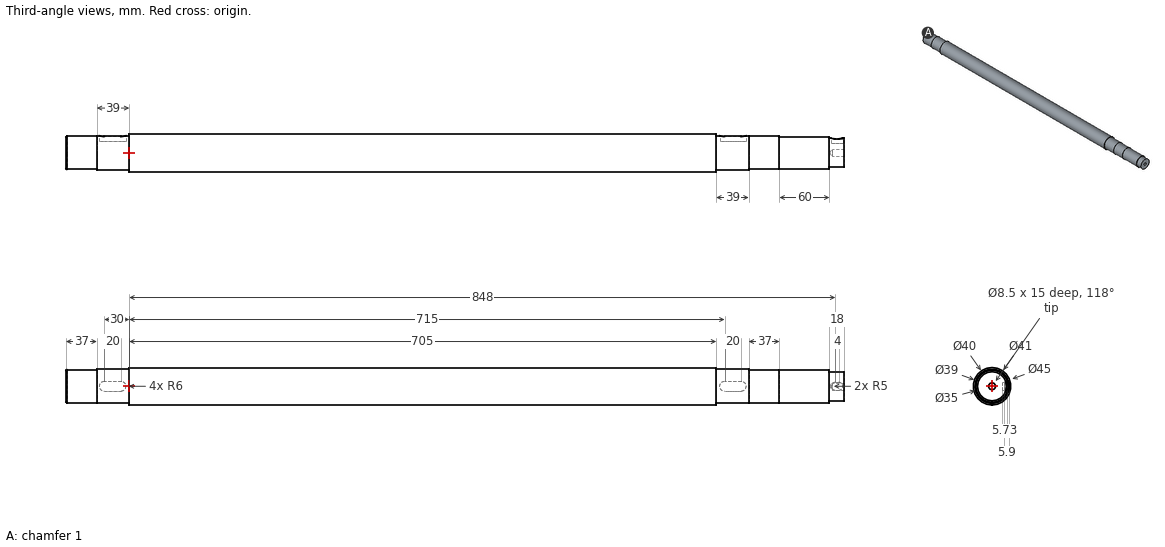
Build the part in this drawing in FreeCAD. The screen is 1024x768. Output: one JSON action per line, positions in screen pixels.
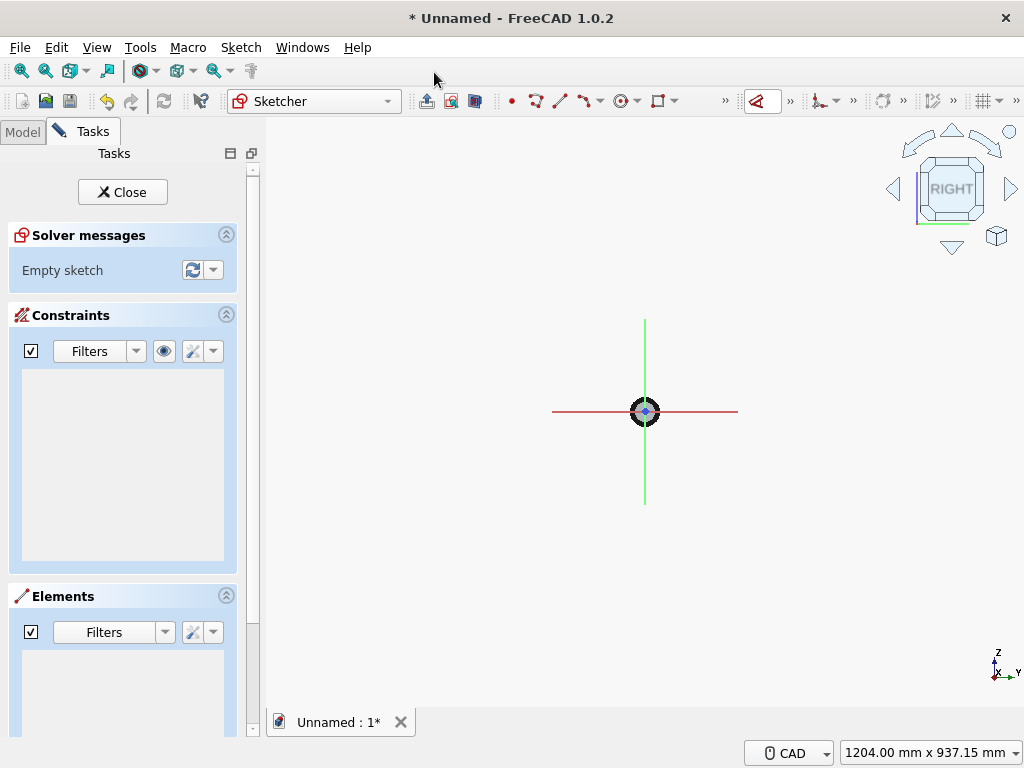
{"action": "scroll", "coordinate": [649, 412], "scroll_direction": "up", "scroll_amount": 15}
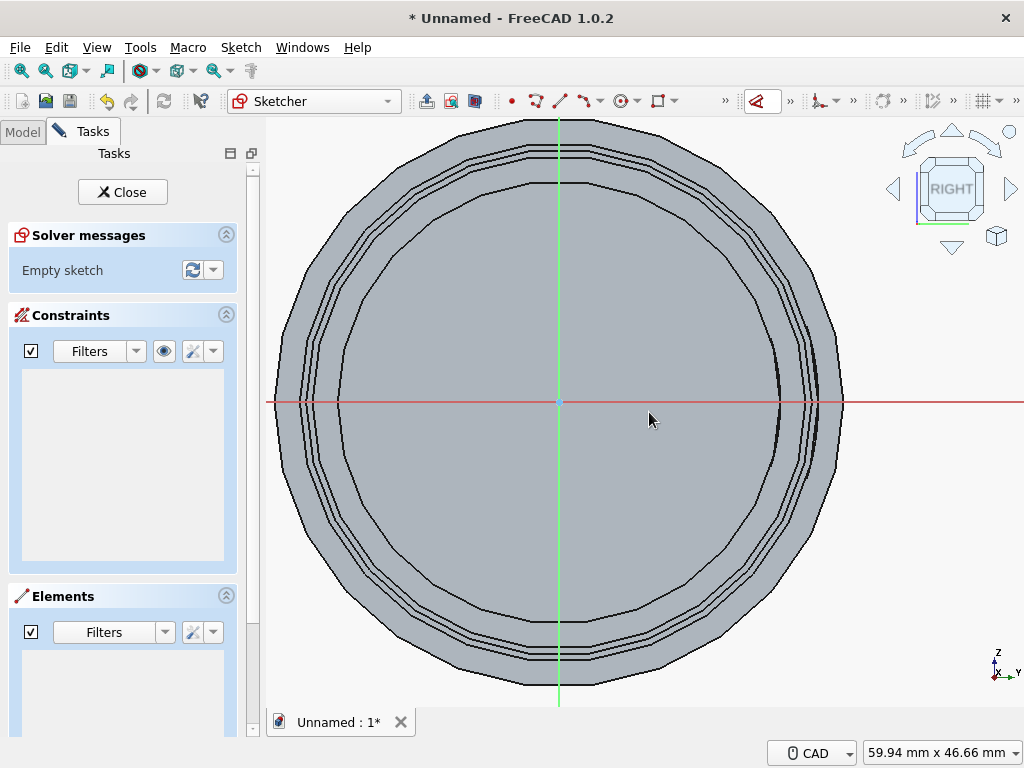
{"action": "scroll", "coordinate": [551, 398], "scroll_direction": "up", "scroll_amount": 6}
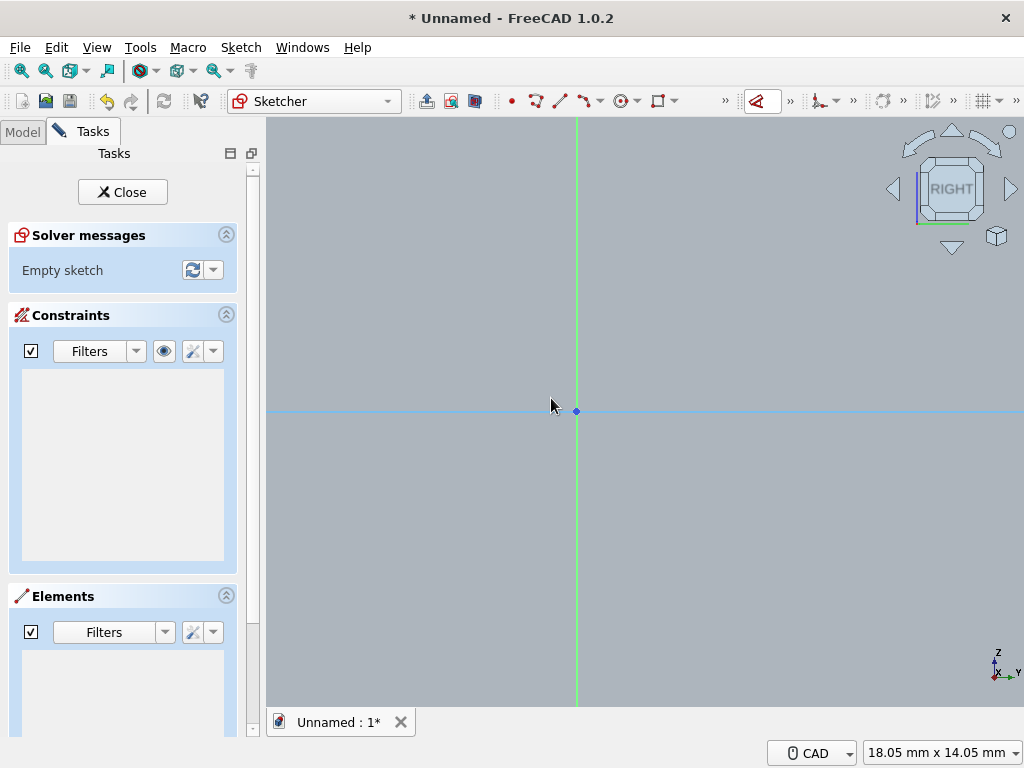
{"action": "left_click", "coordinate": [622, 102]}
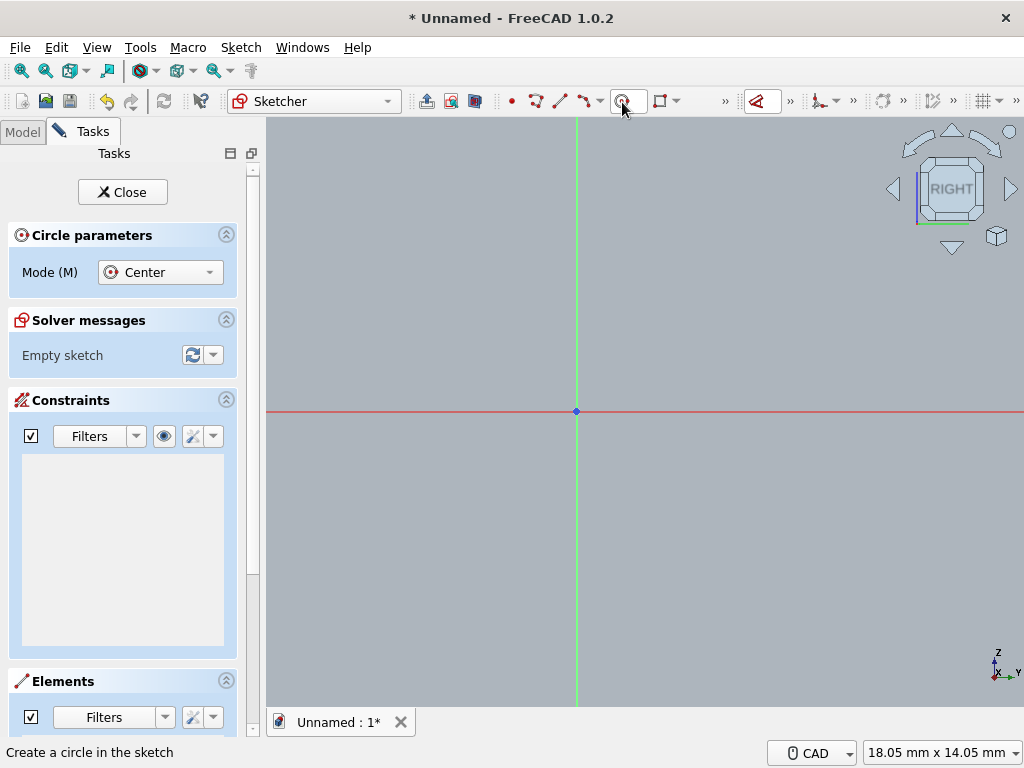
{"action": "left_click", "coordinate": [577, 412]}
{"action": "mouse_move", "coordinate": [703, 285]}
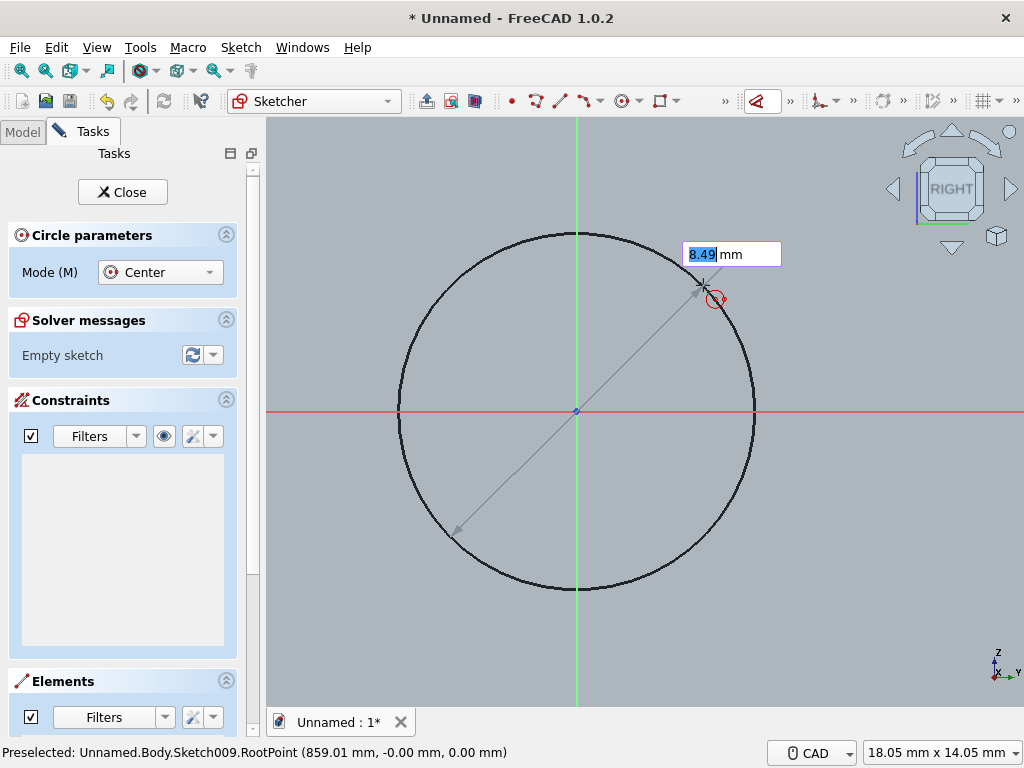
{"action": "type", "text": "8.5"}
{"action": "key", "text": "Return"}
{"action": "key", "text": "Escape"}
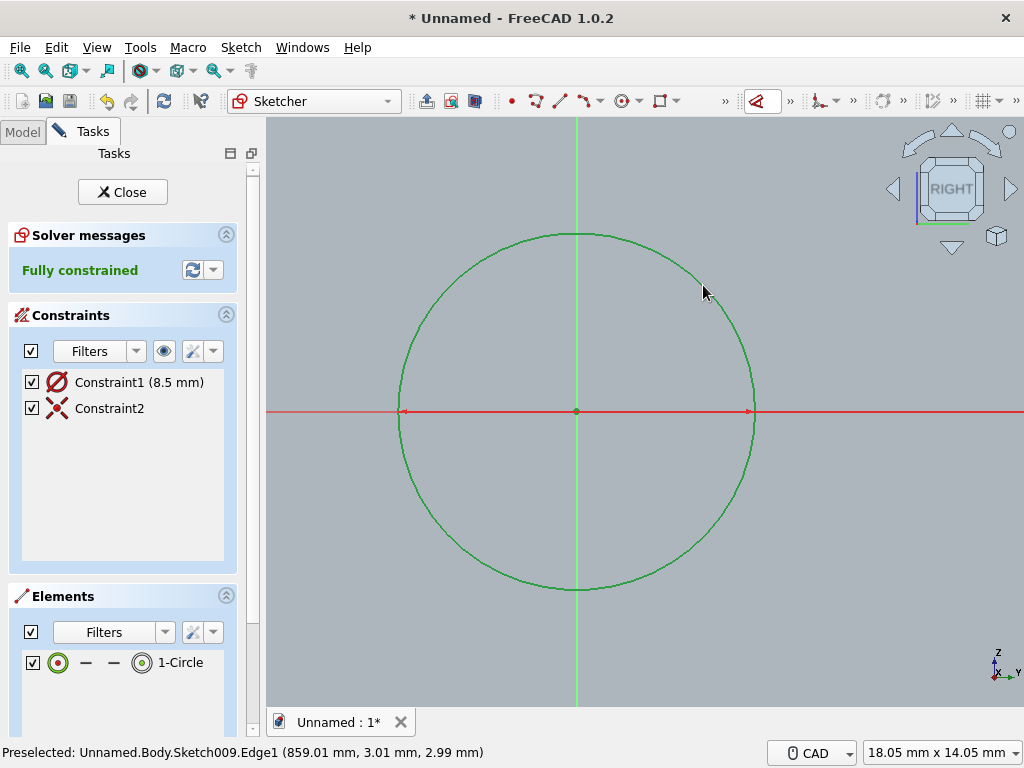
{"action": "left_click", "coordinate": [123, 192]}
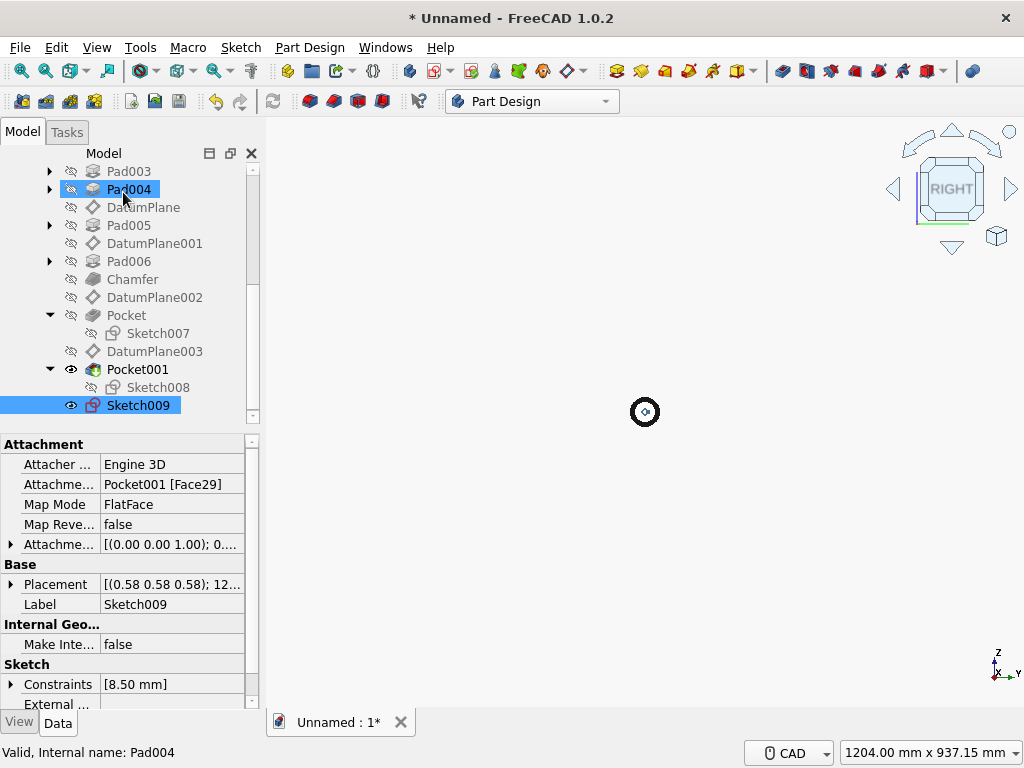
{"action": "left_click", "coordinate": [808, 72]}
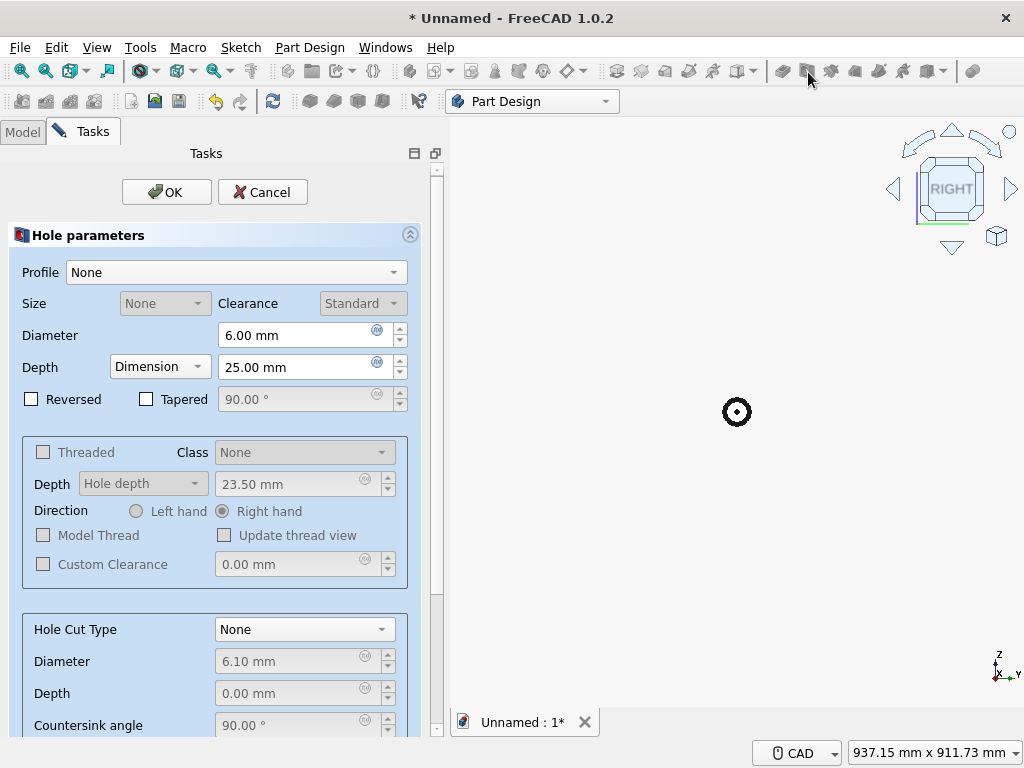
{"action": "triple_click", "coordinate": [305, 335]}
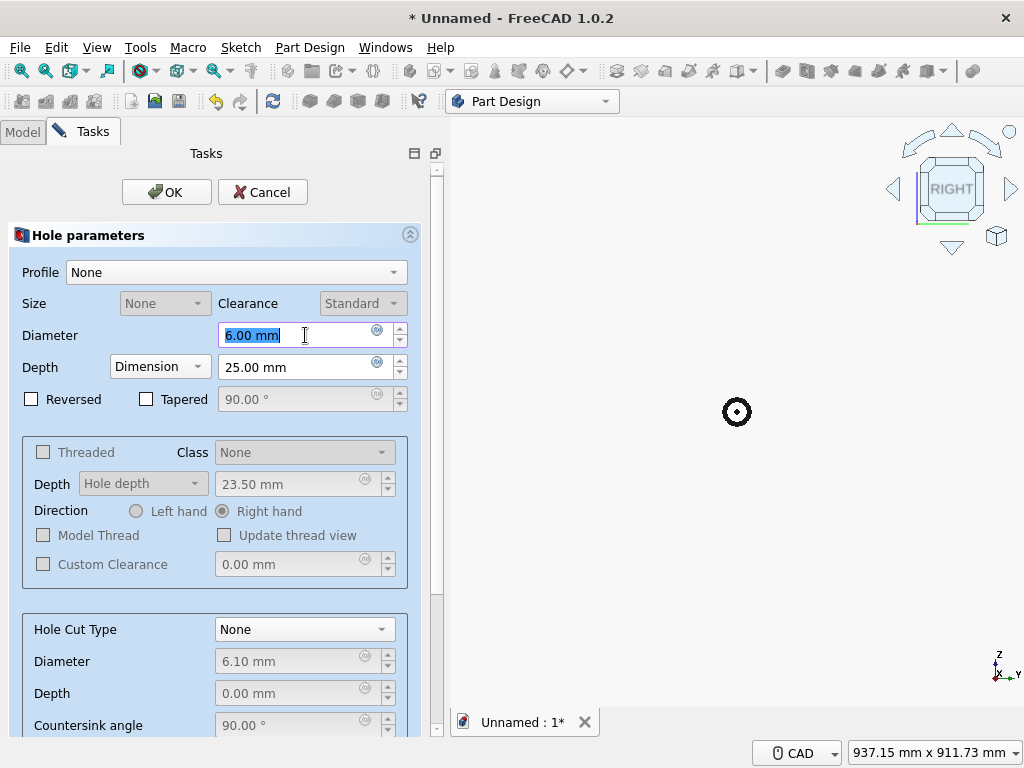
{"action": "type", "text": "8.5"}
{"action": "key", "text": "Tab"}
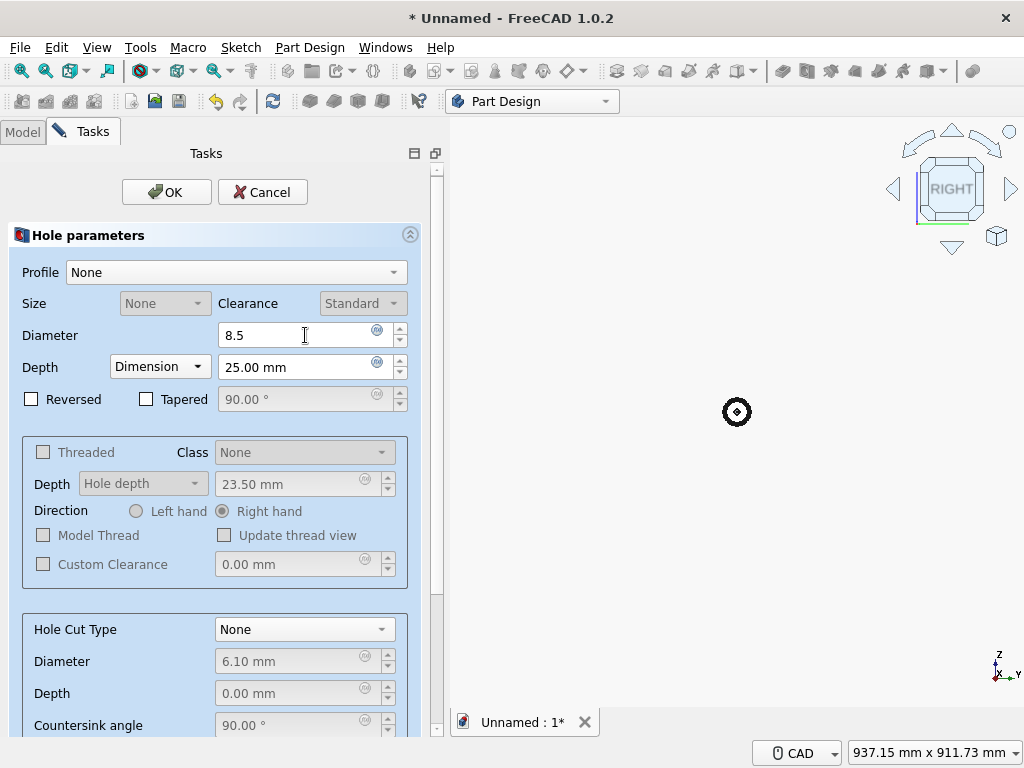
{"action": "triple_click", "coordinate": [305, 367]}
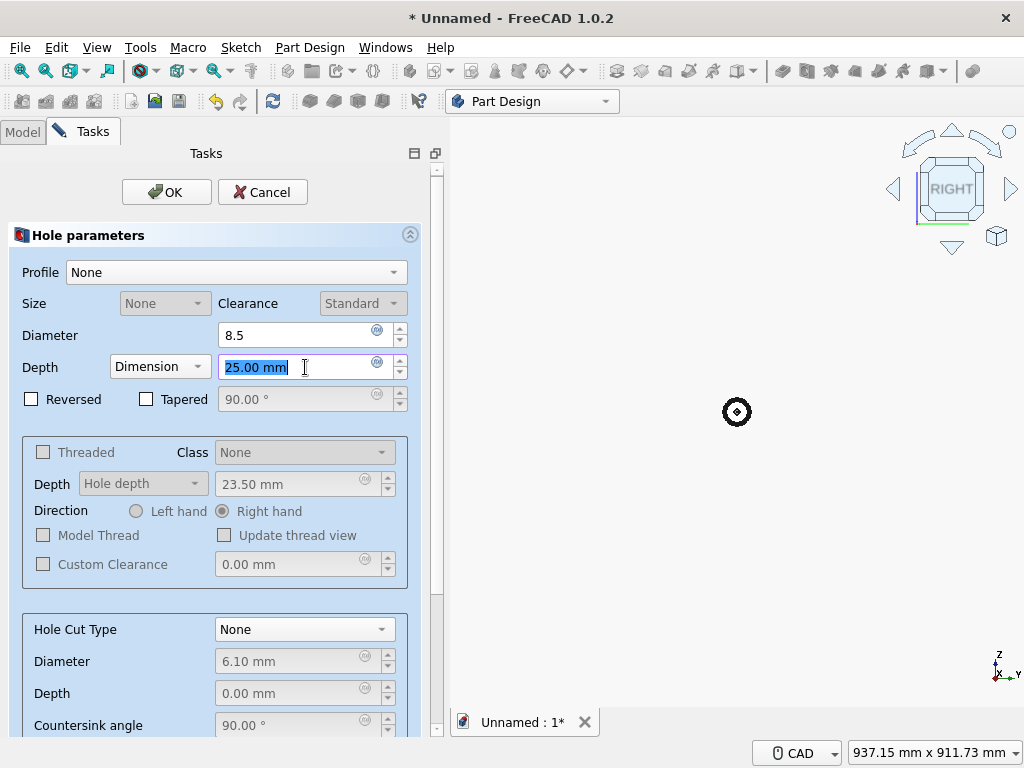
{"action": "type", "text": "15"}
{"action": "key", "text": "Tab"}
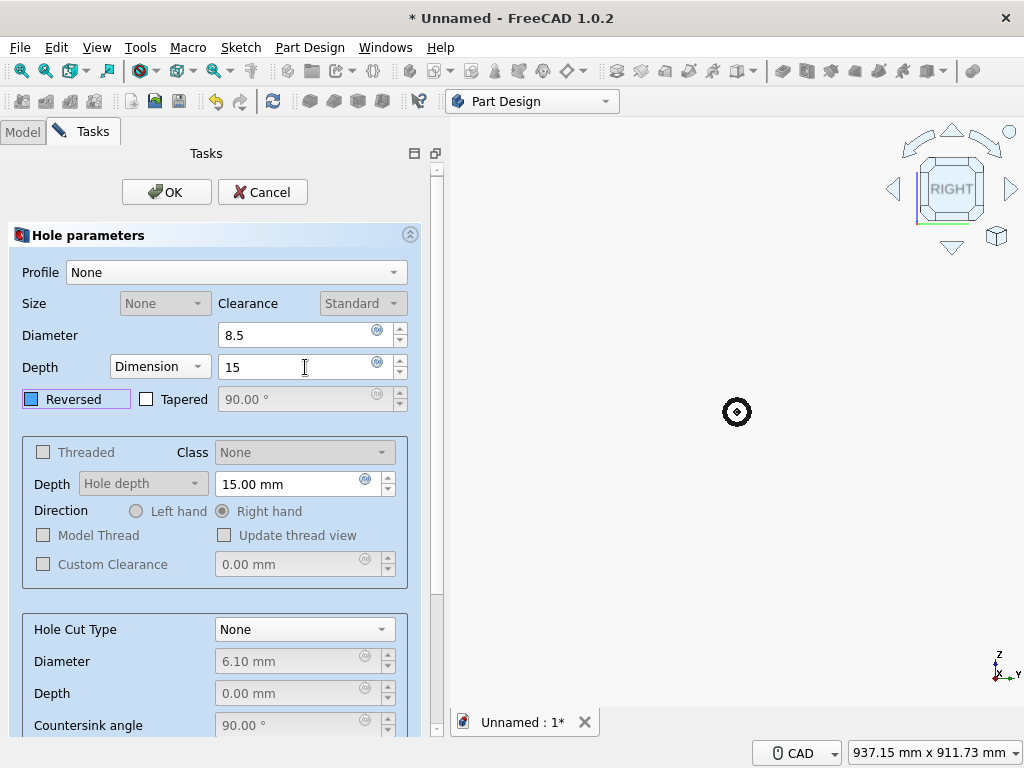
{"action": "left_click", "coordinate": [167, 192]}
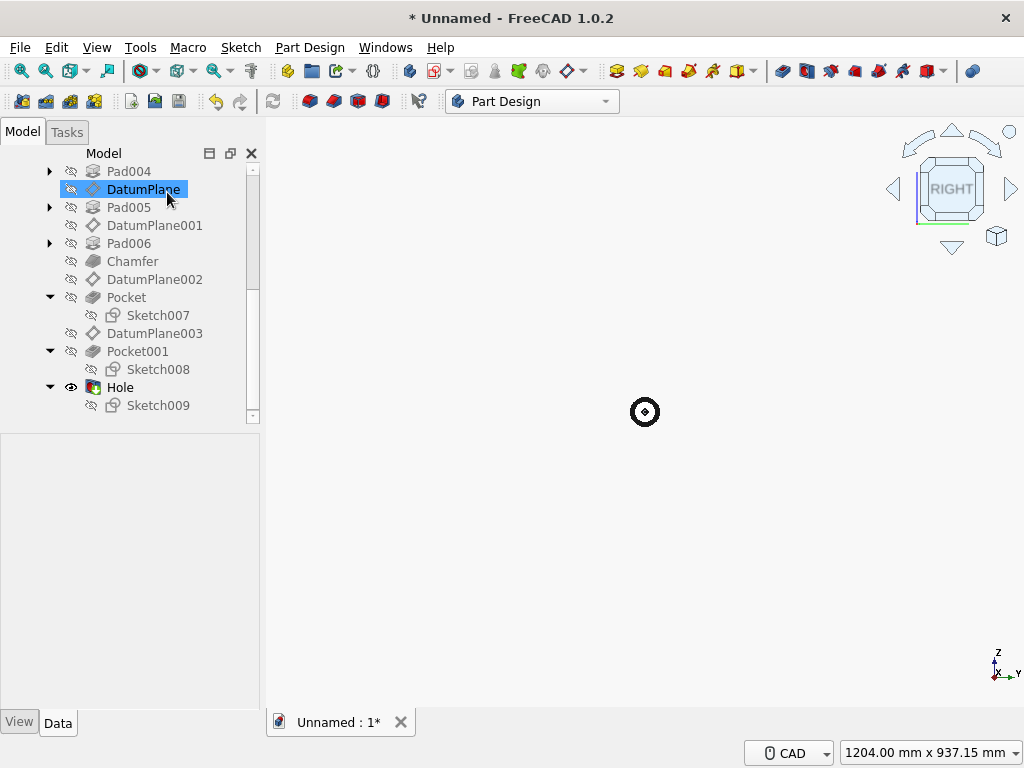
{"action": "key", "text": "0"}